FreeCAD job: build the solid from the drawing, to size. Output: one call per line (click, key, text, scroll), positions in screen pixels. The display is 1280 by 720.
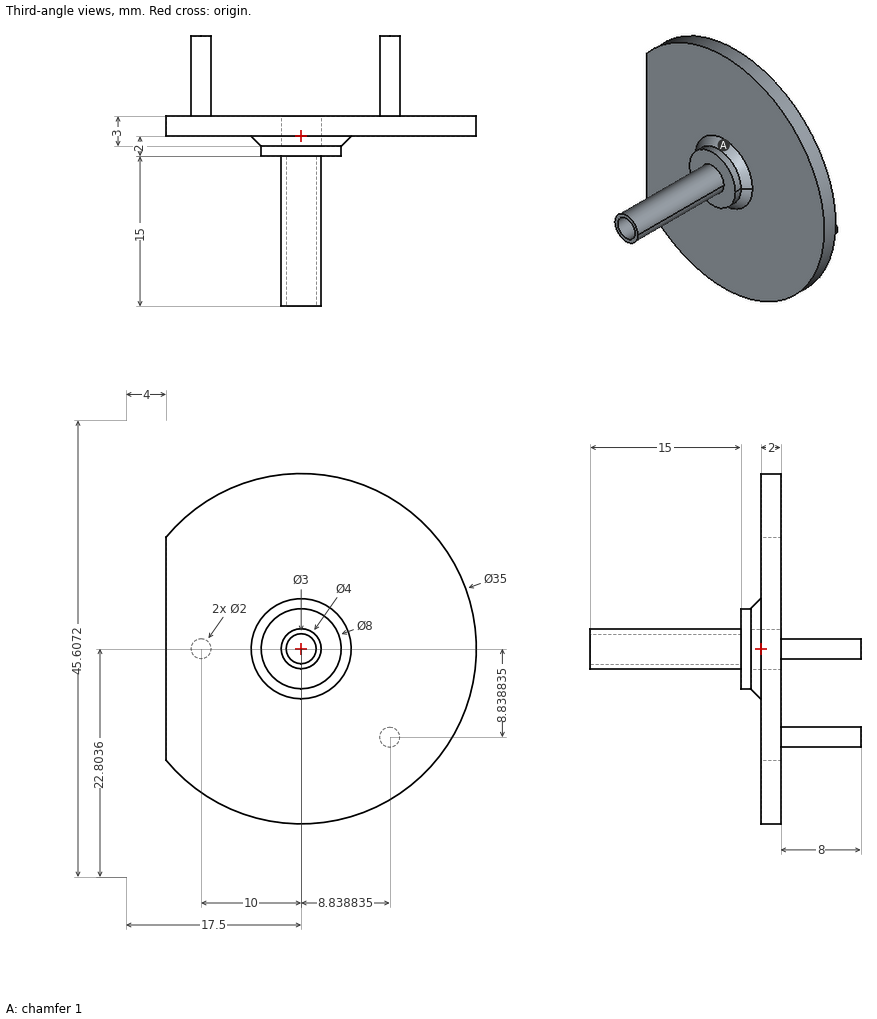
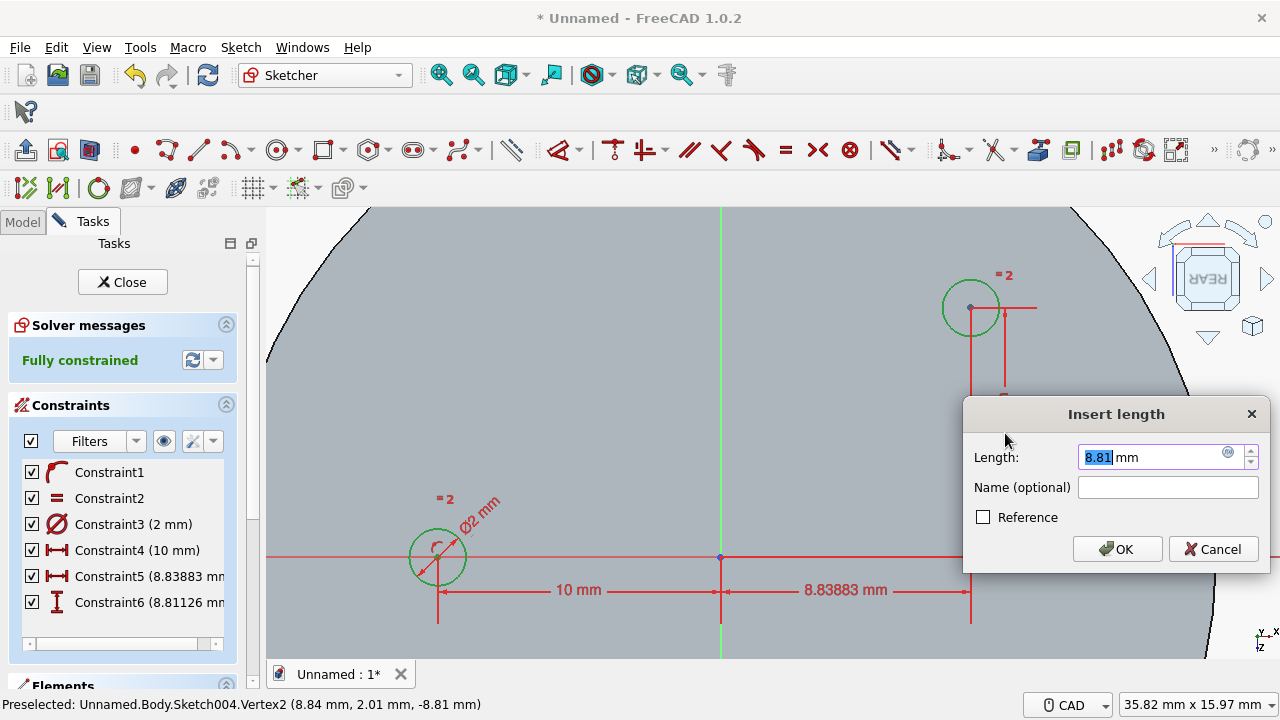
text(8.838835)
key(Return)
key(Escape)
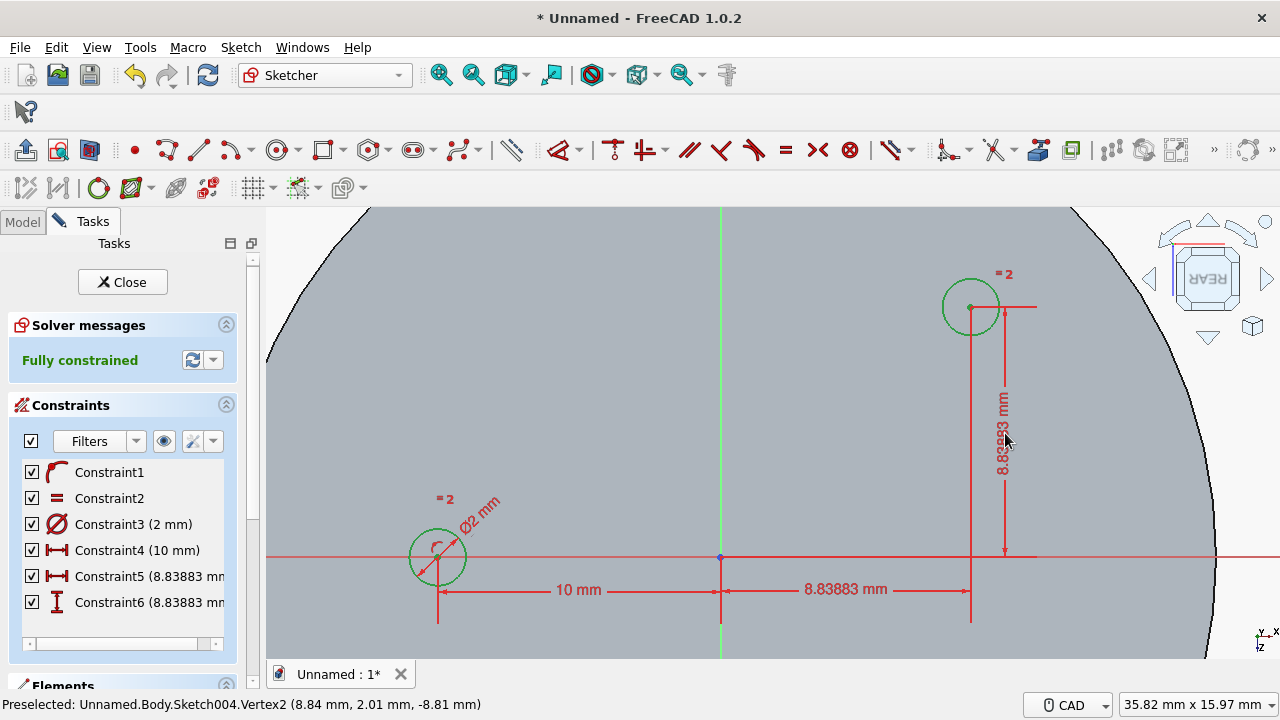
click(123, 282)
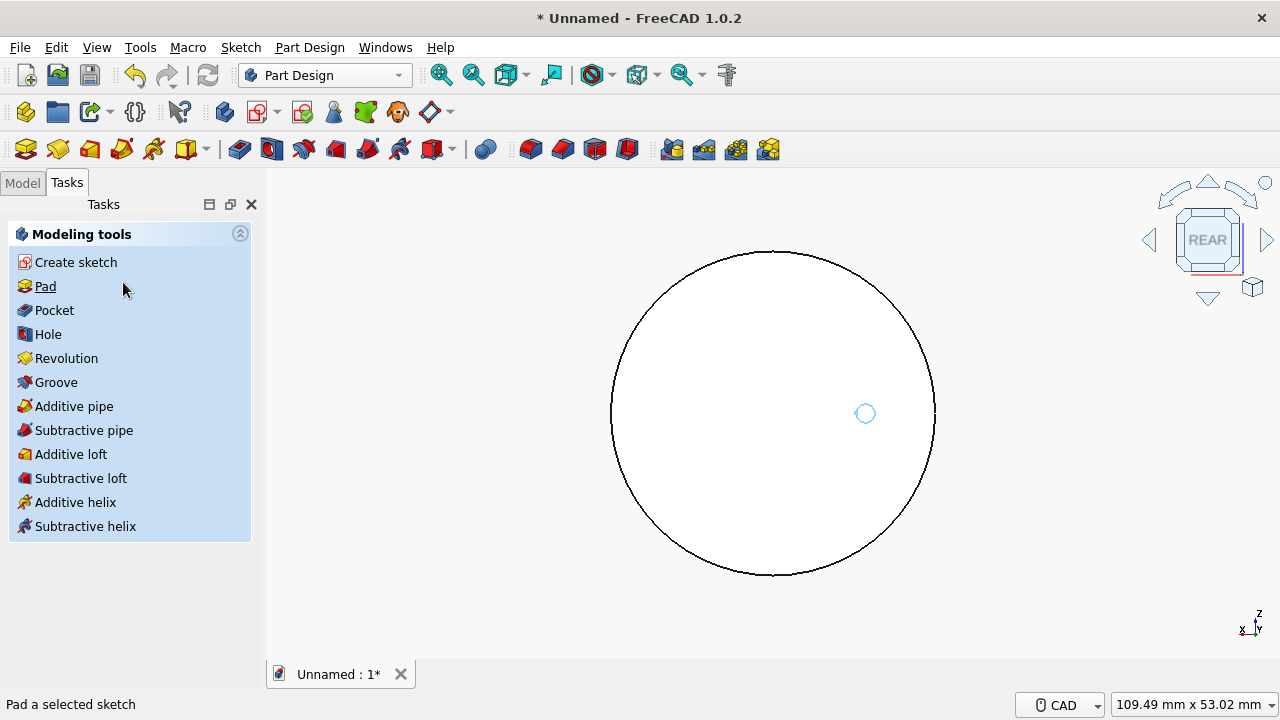
click(26, 150)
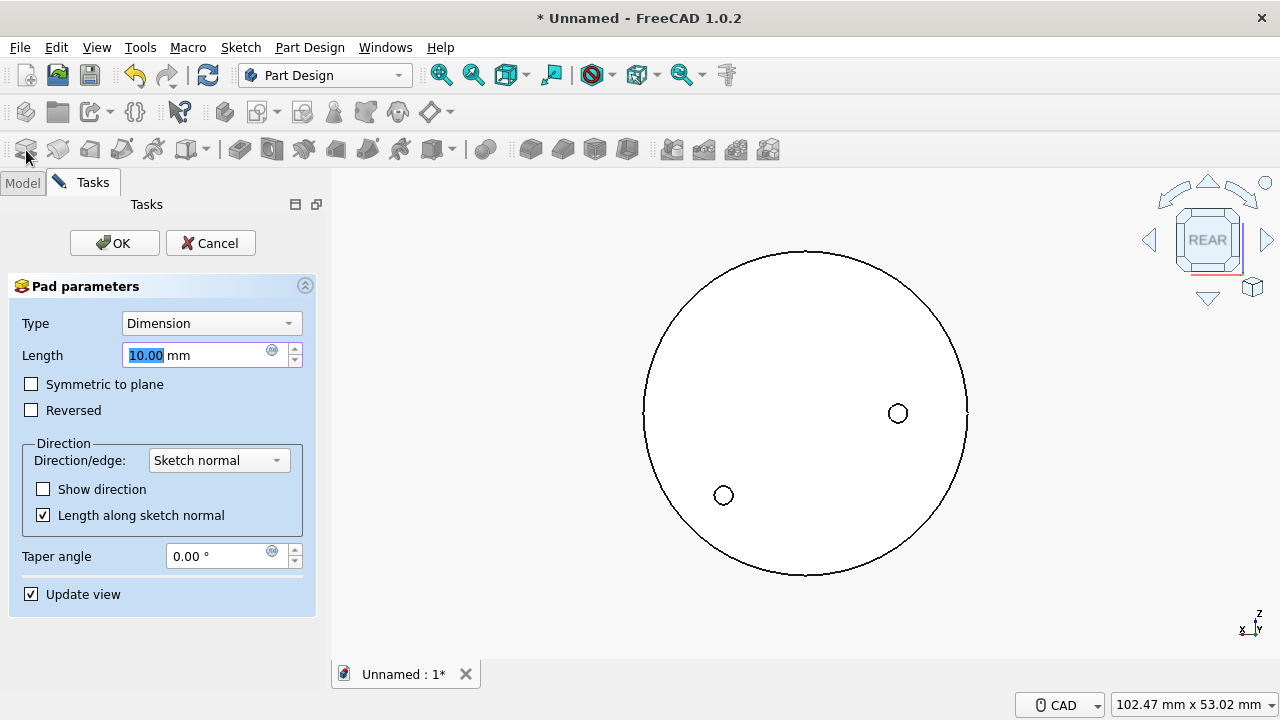
text(8)
key(Tab)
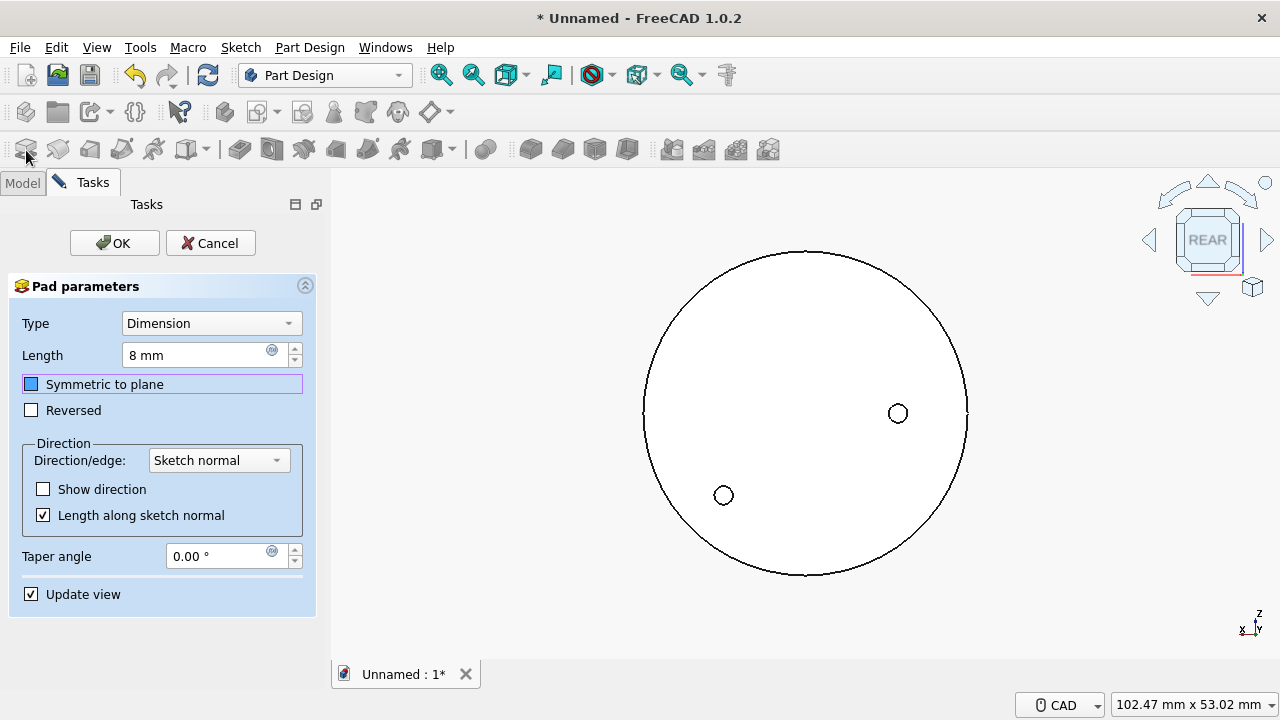
click(115, 243)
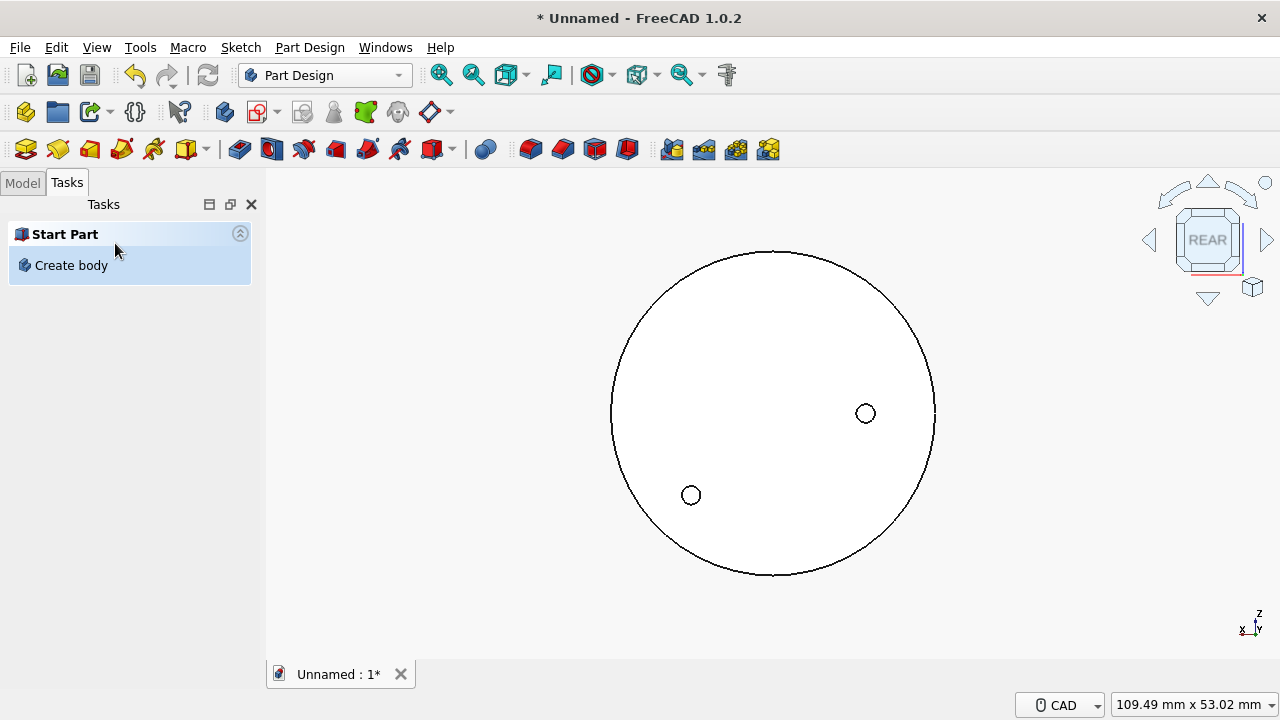
click(727, 366)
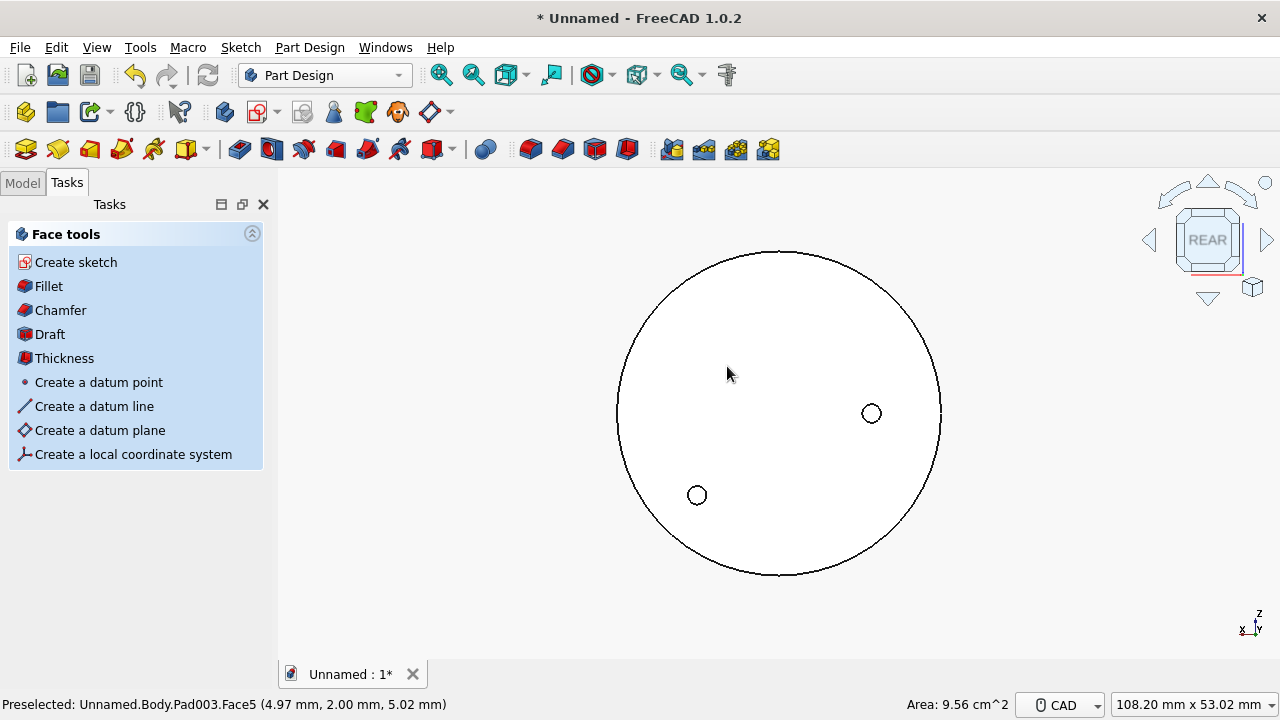
click(258, 112)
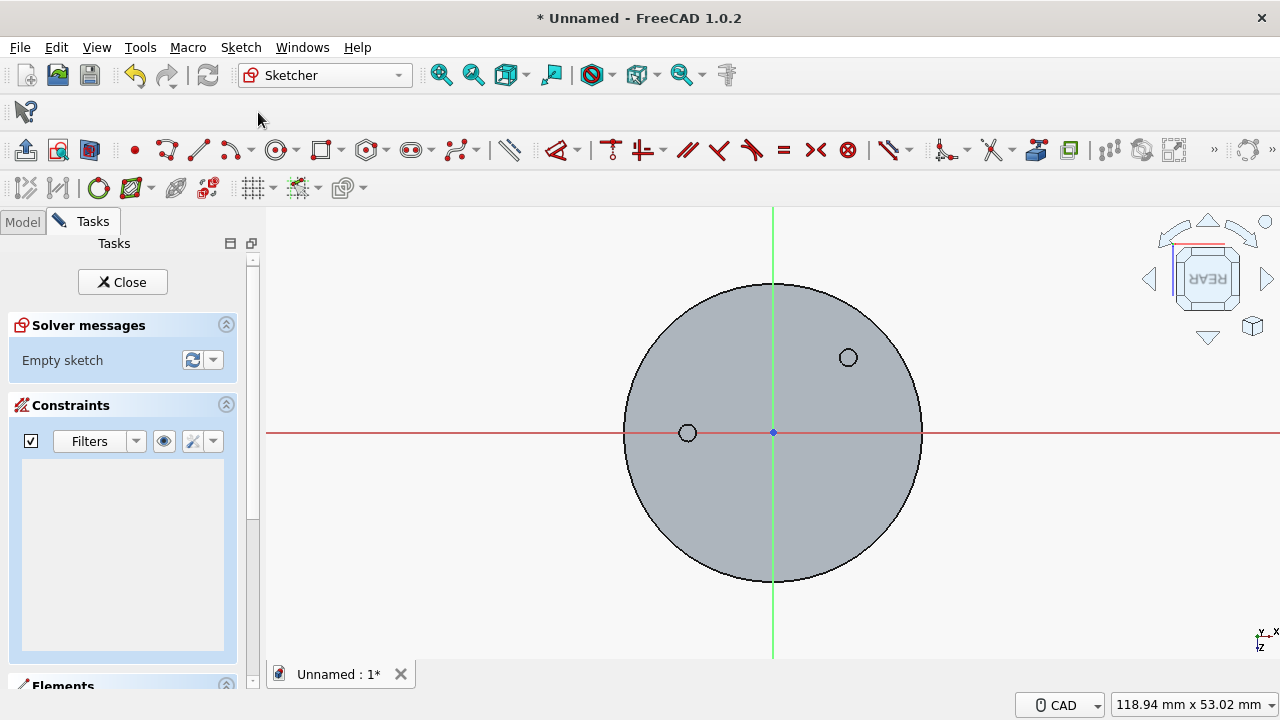
scroll(717, 433, down, 2)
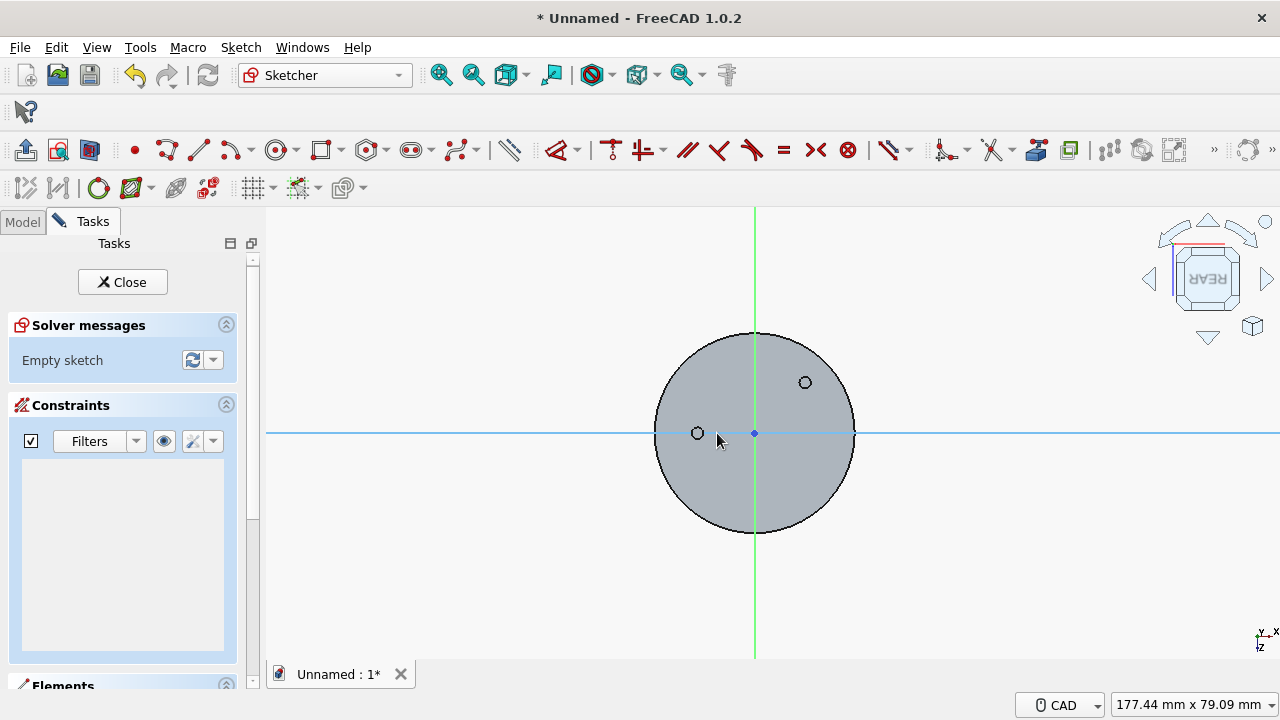
click(322, 150)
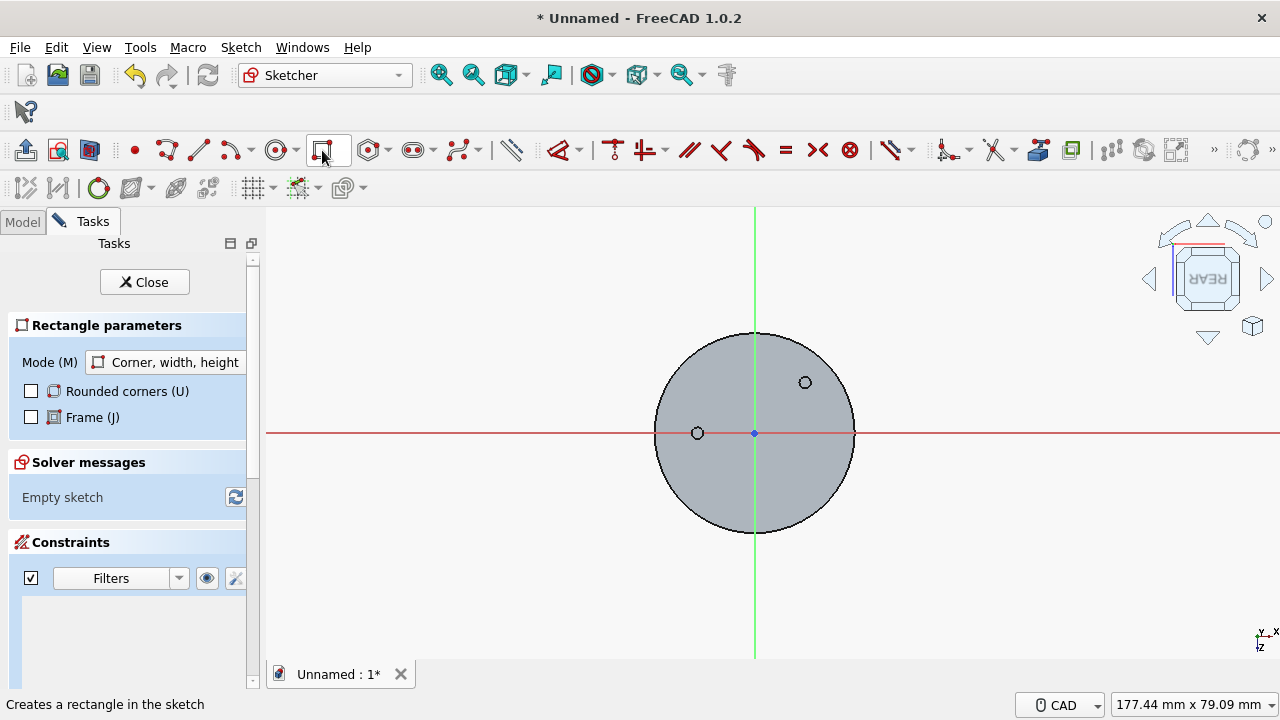
click(655, 303)
click(678, 563)
key(Escape)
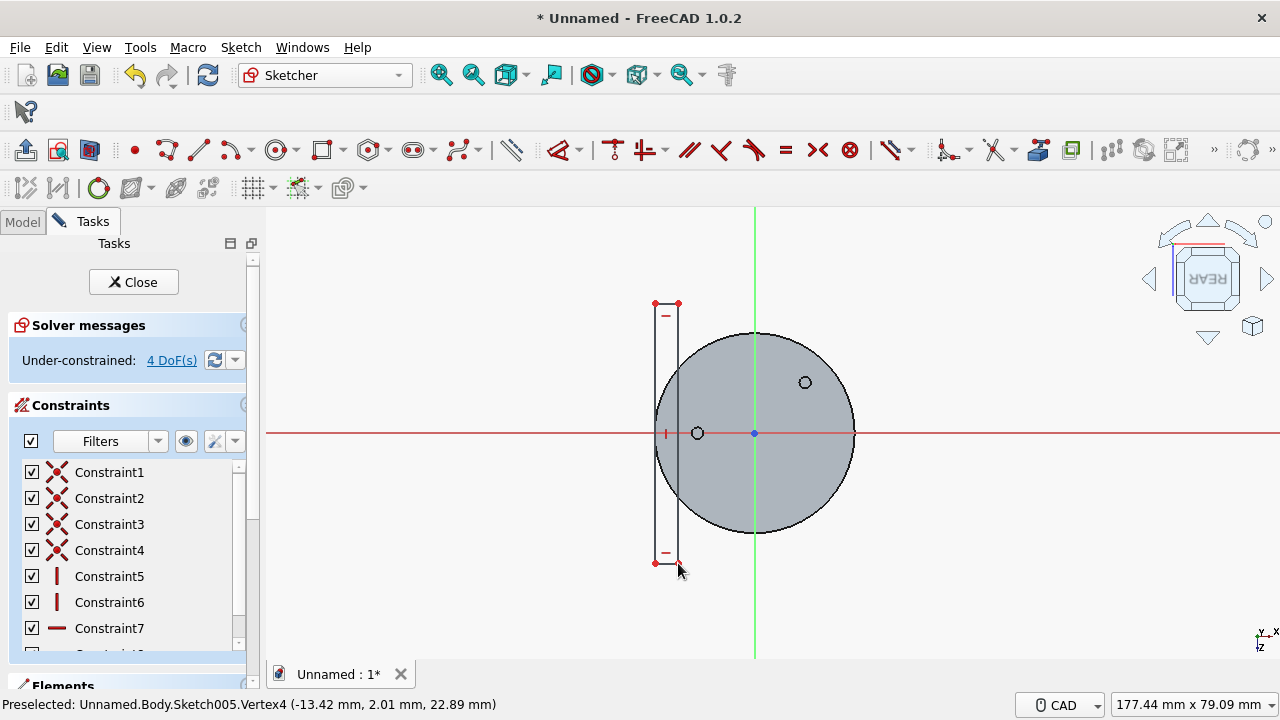
click(558, 150)